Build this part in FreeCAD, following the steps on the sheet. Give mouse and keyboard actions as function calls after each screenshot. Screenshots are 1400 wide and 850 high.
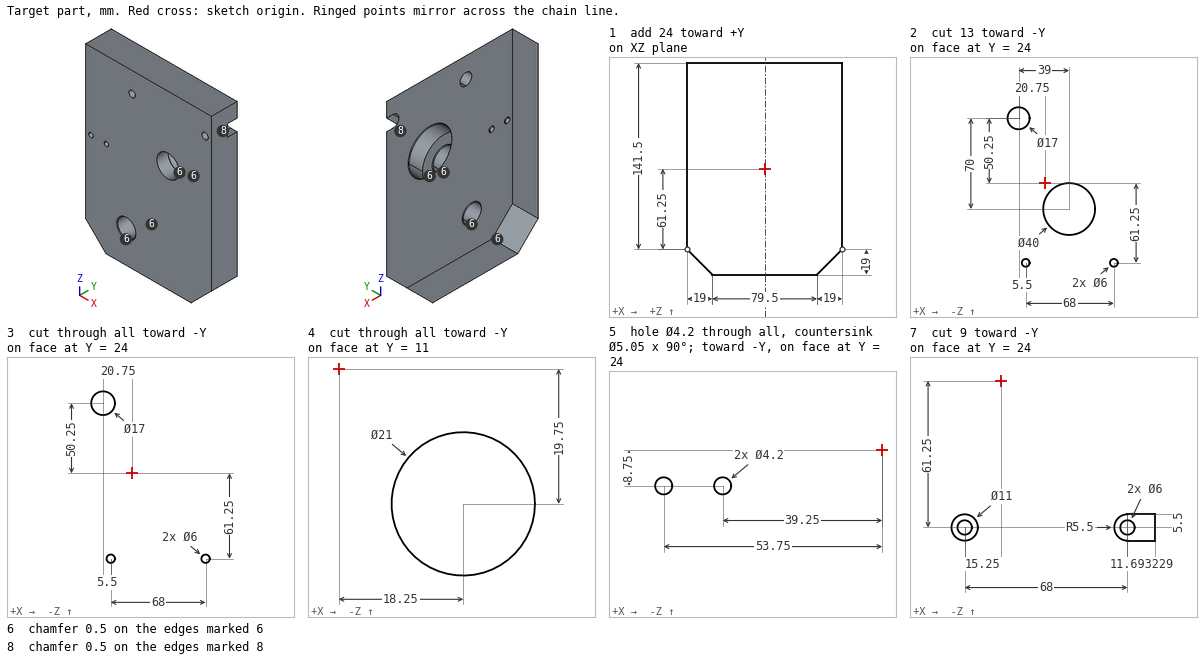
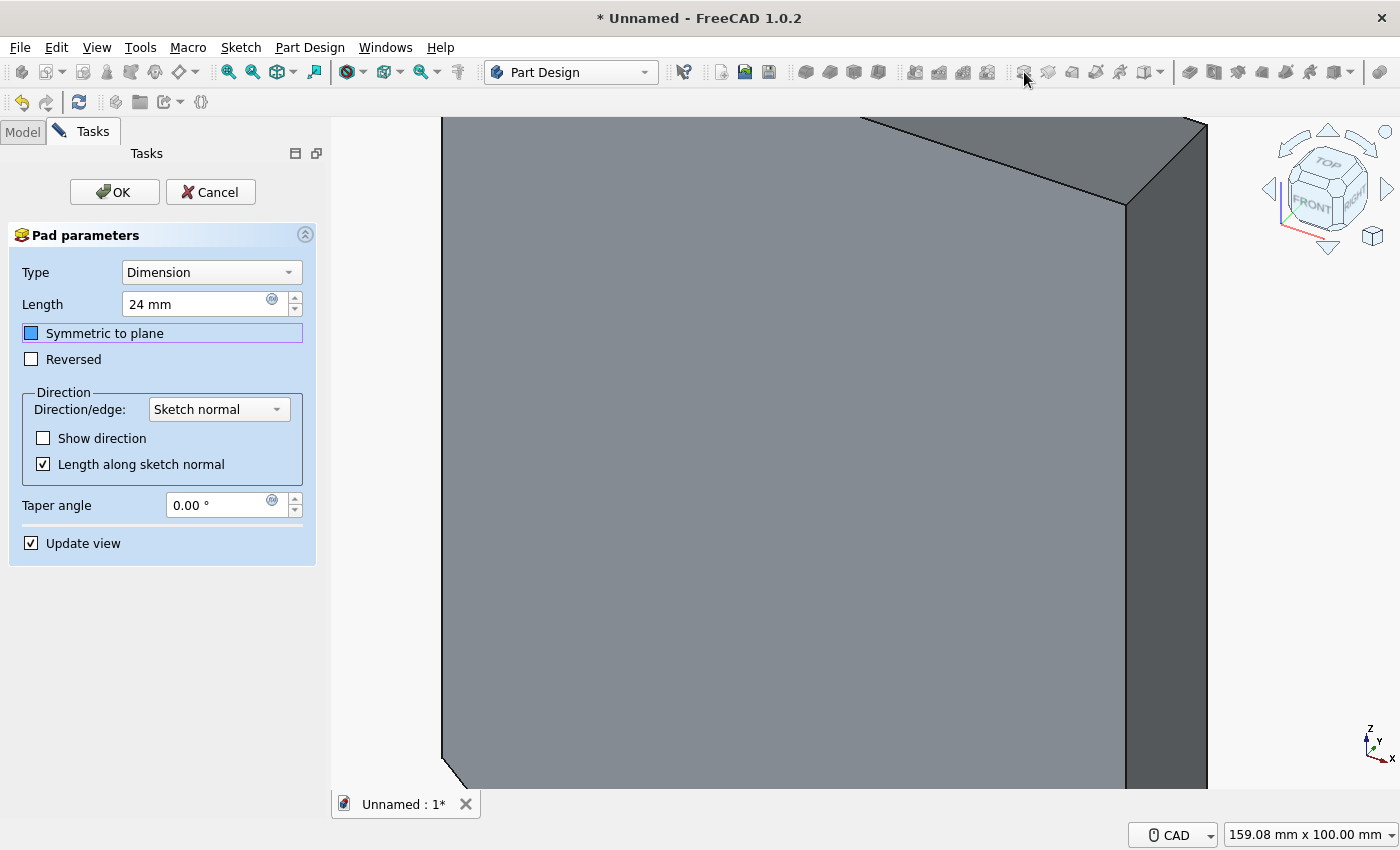
click(30, 359)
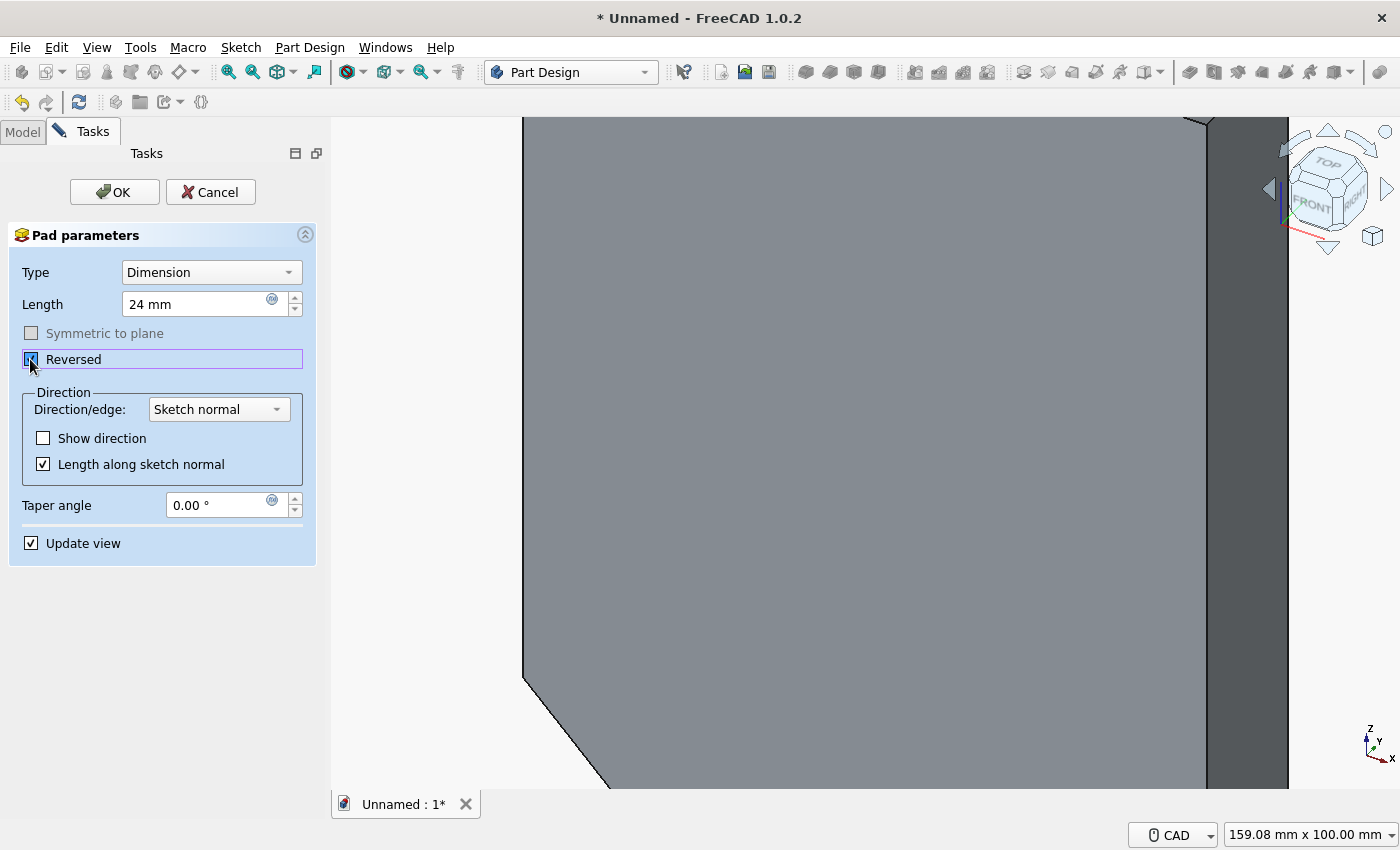
click(115, 192)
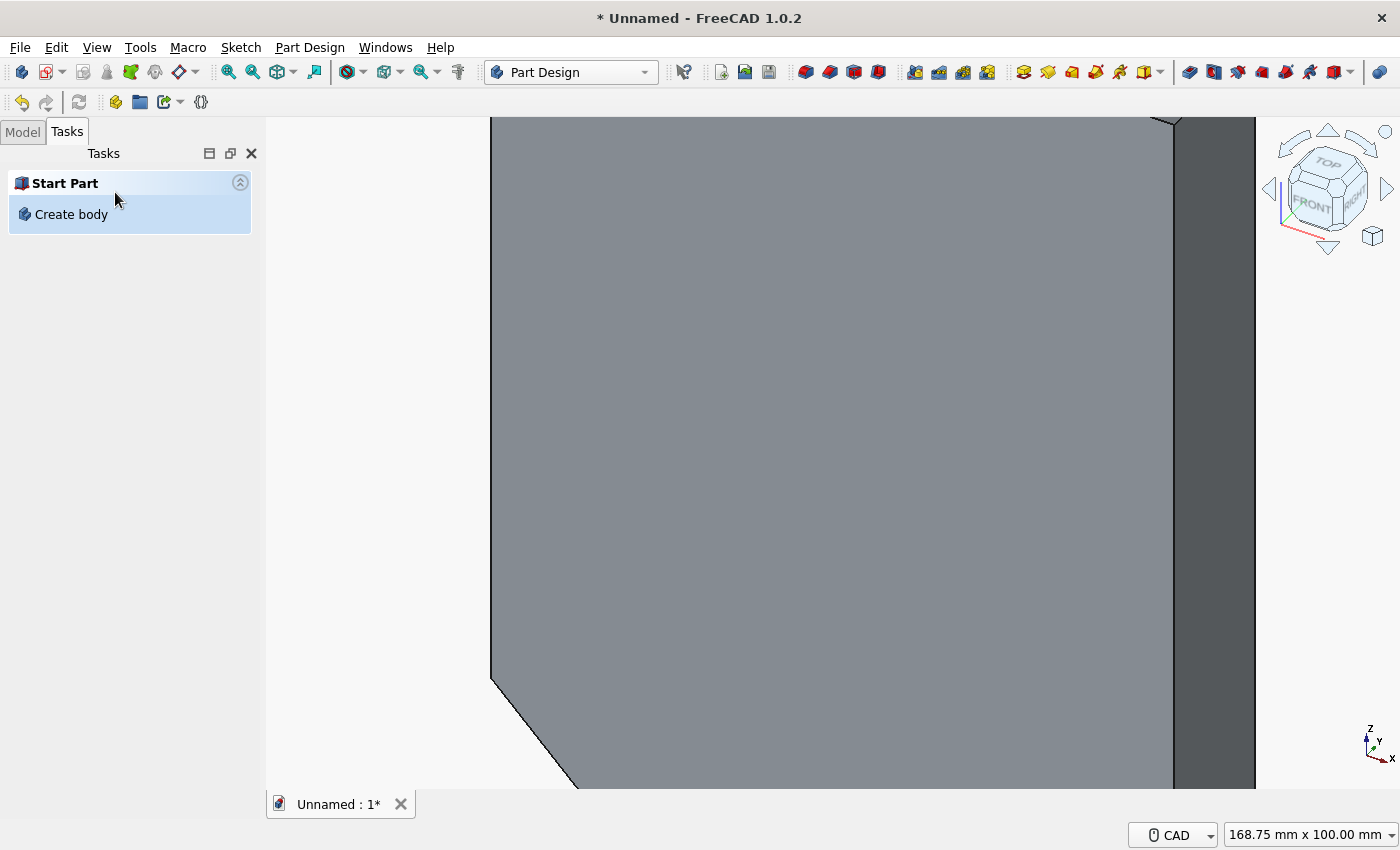
key(v)
key(f)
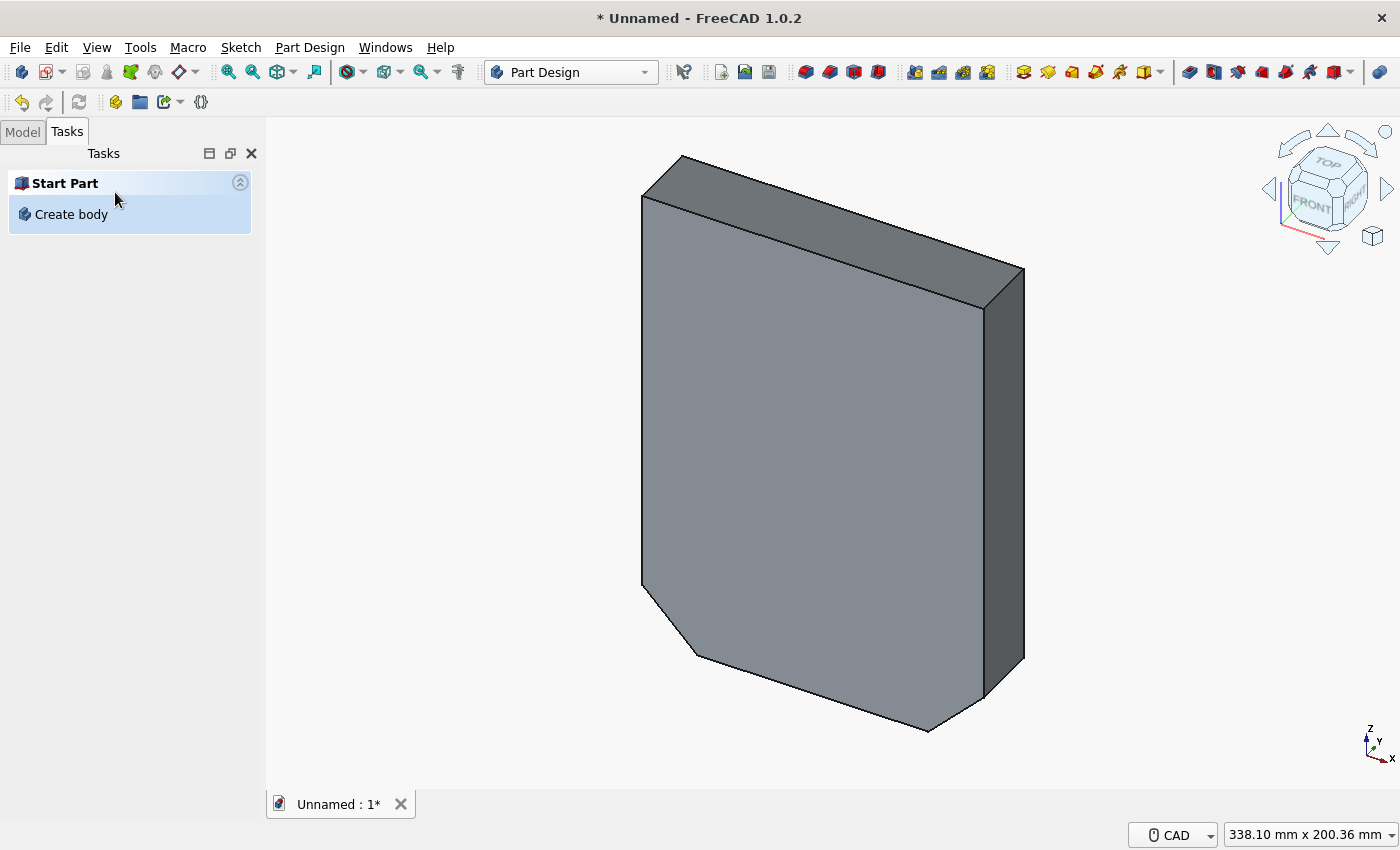
key(4)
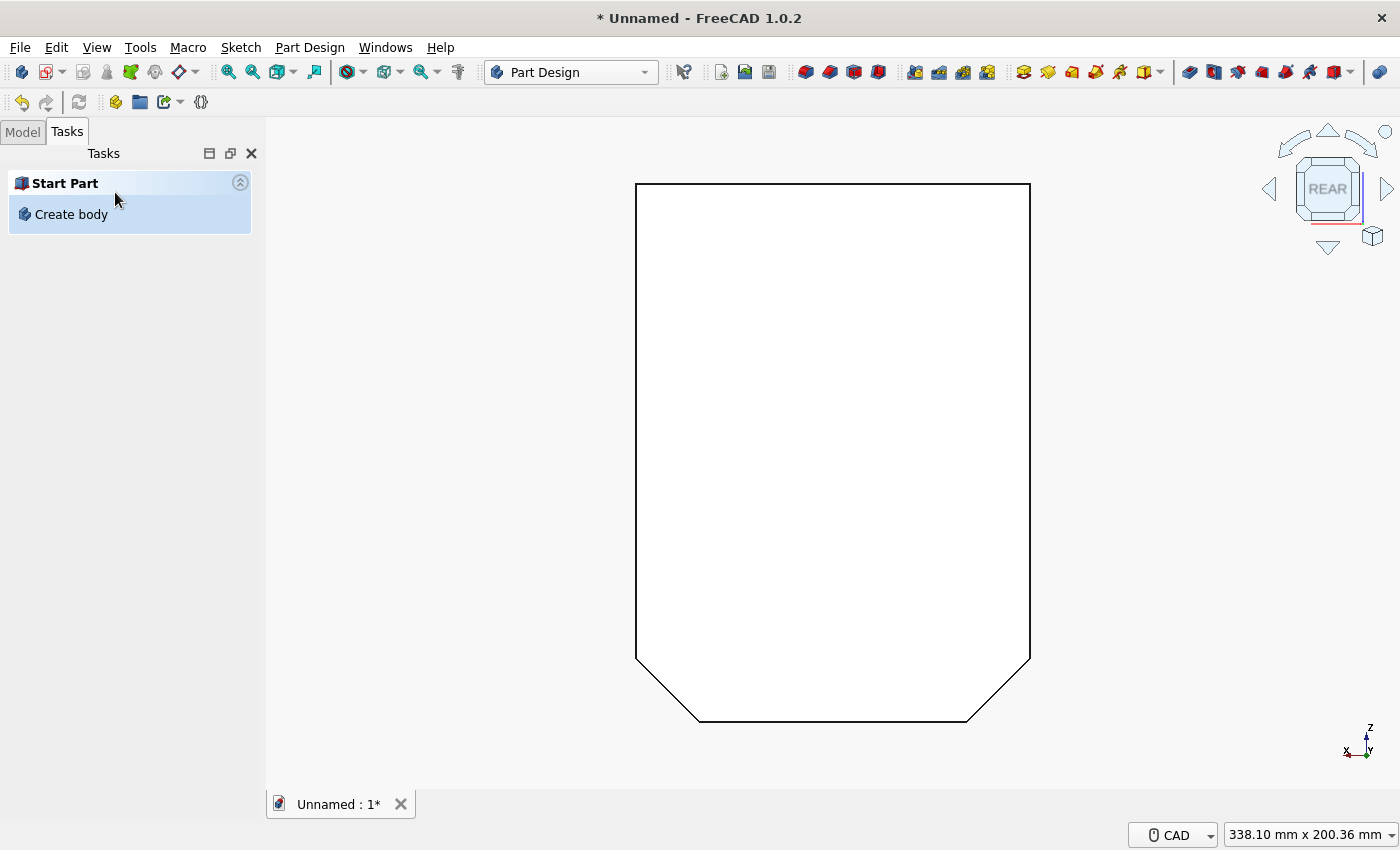
click(833, 452)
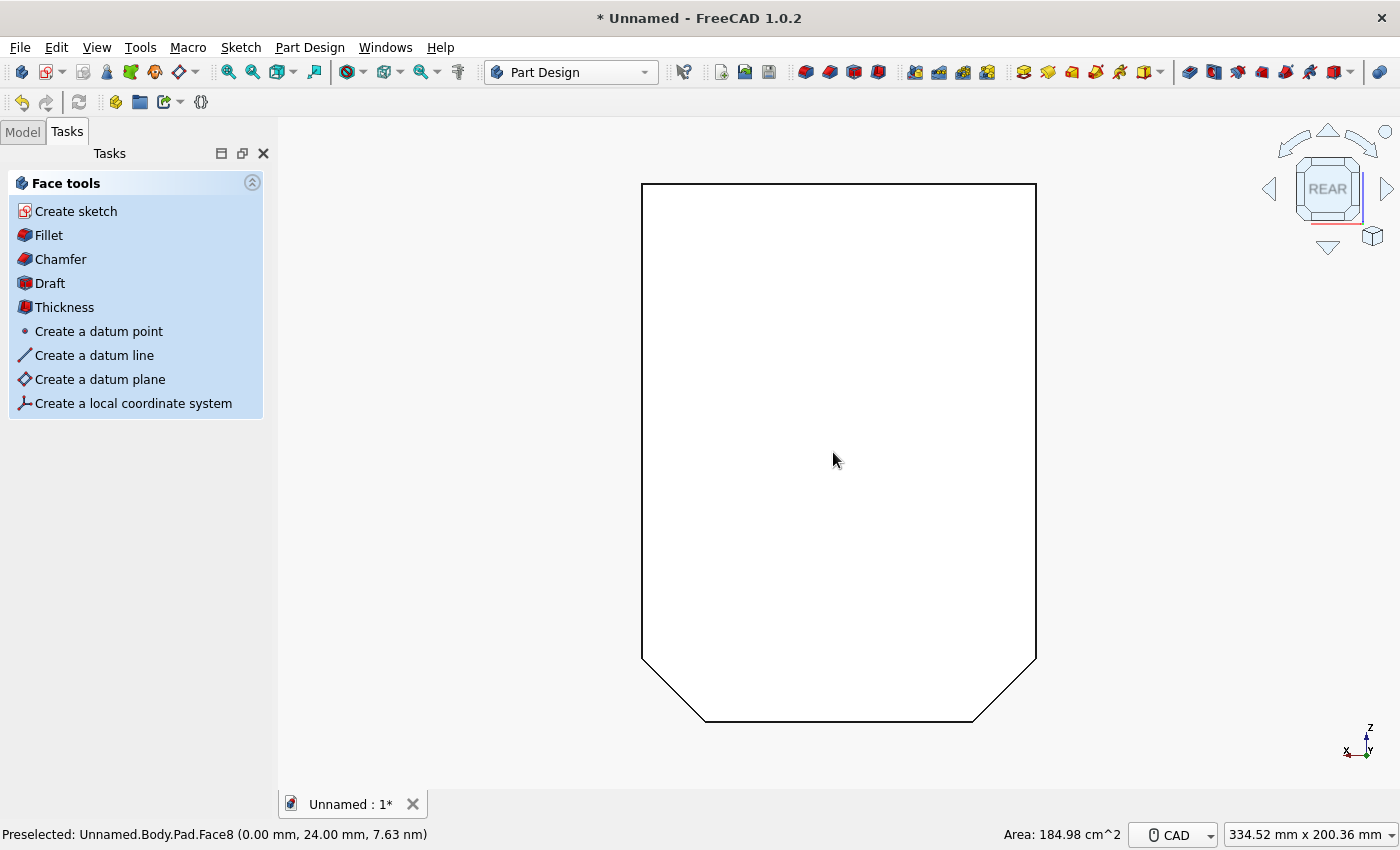
click(46, 72)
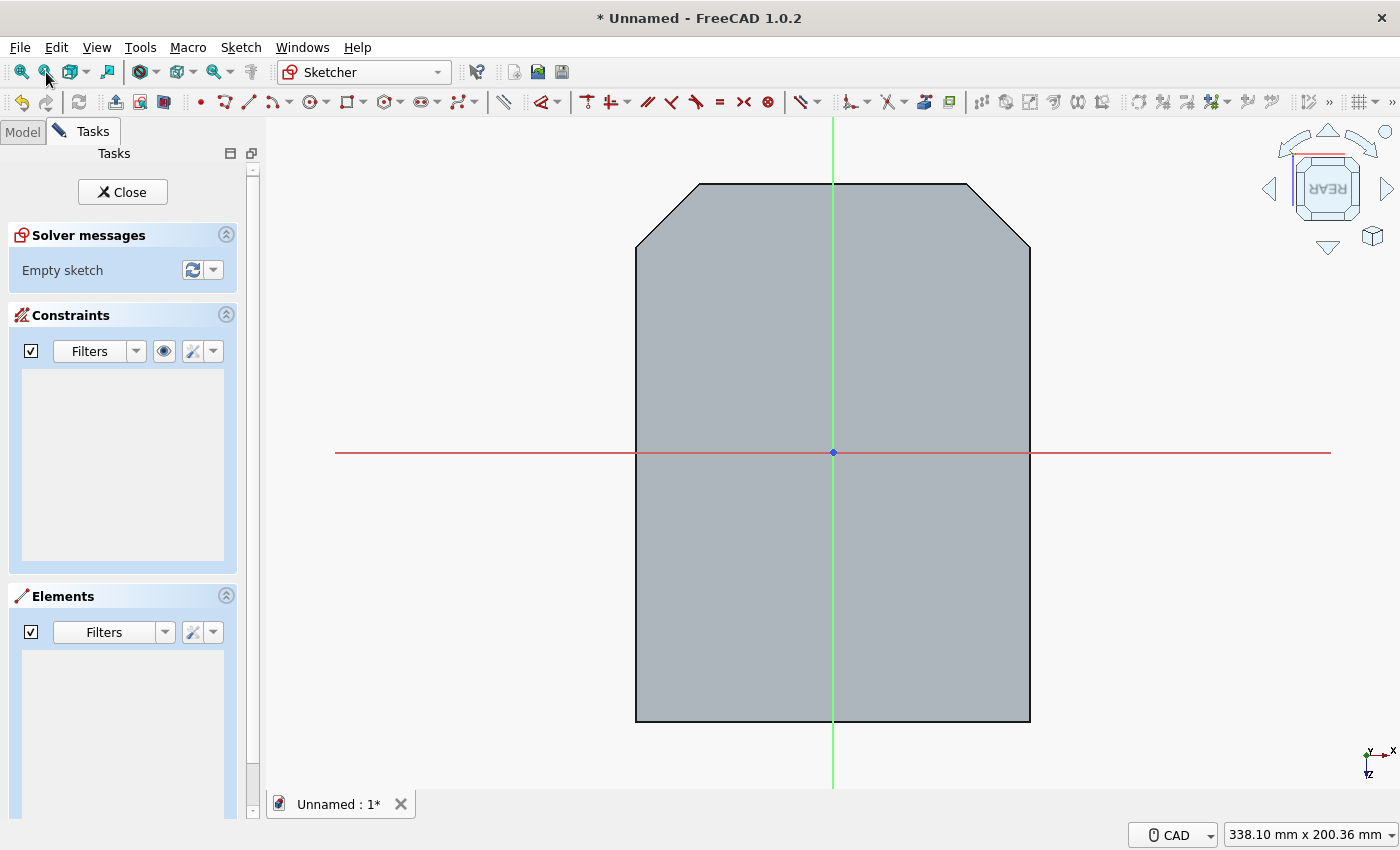
key(g)
key(c)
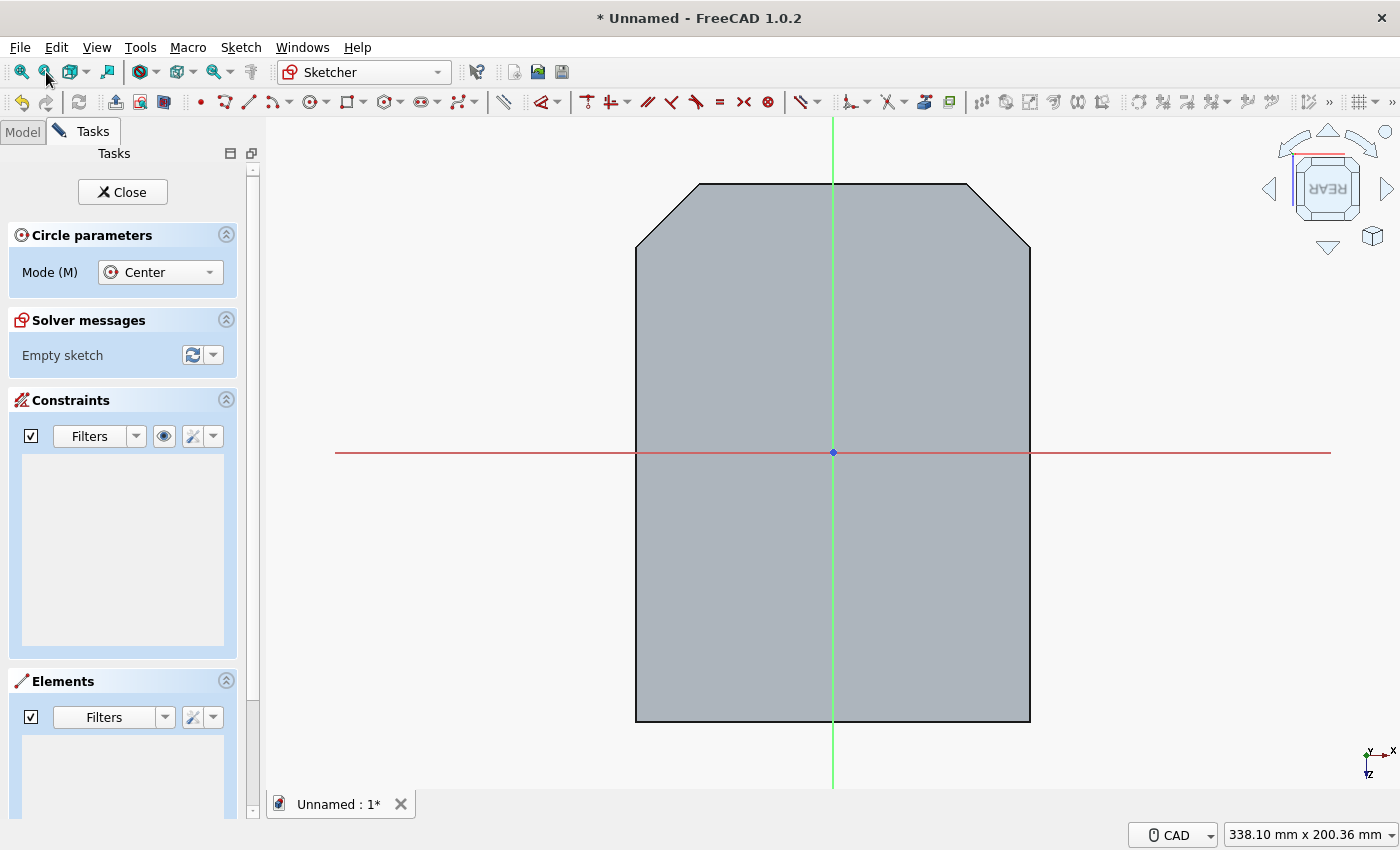
click(763, 284)
move(784, 264)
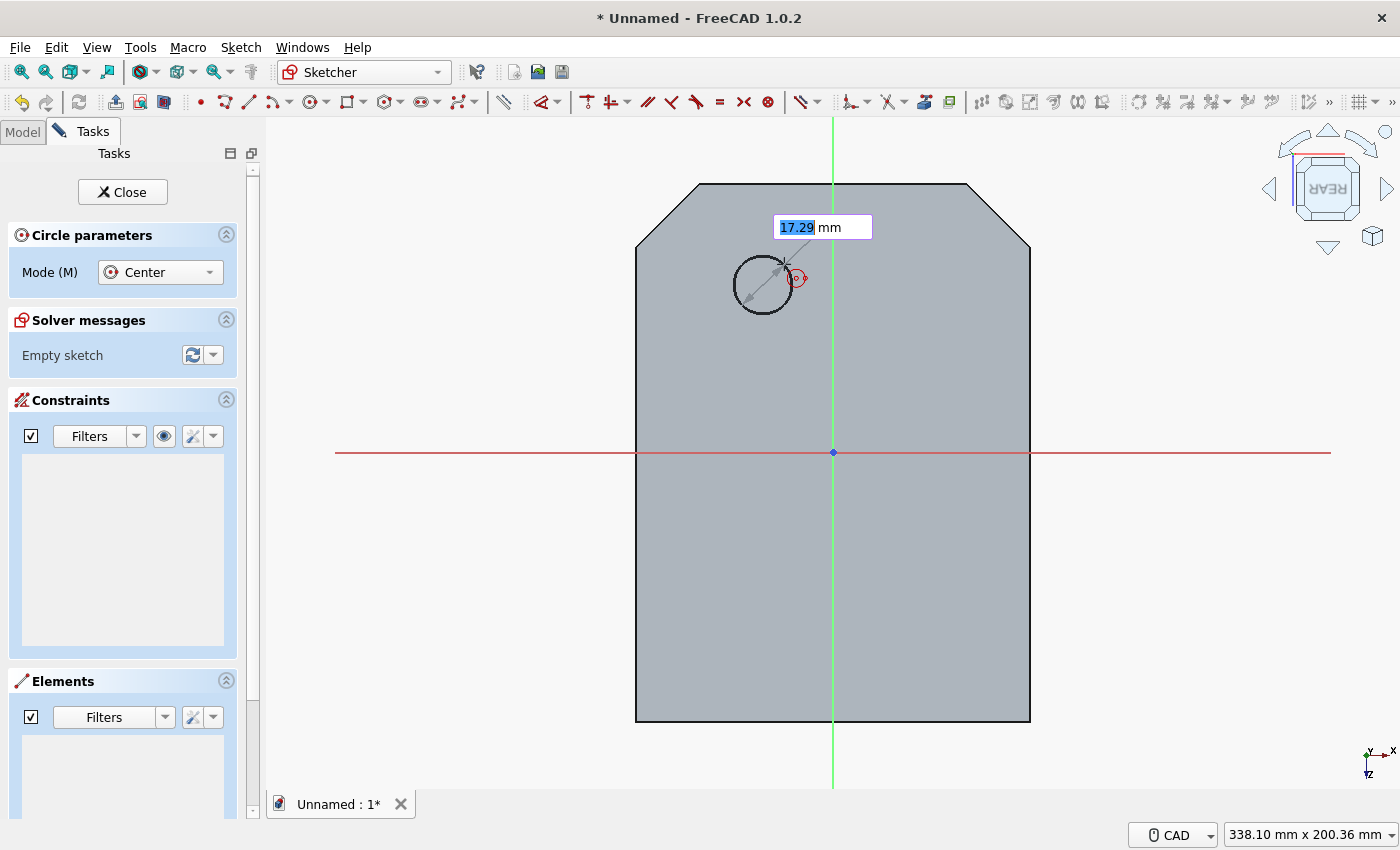
text(17)
key(Return)